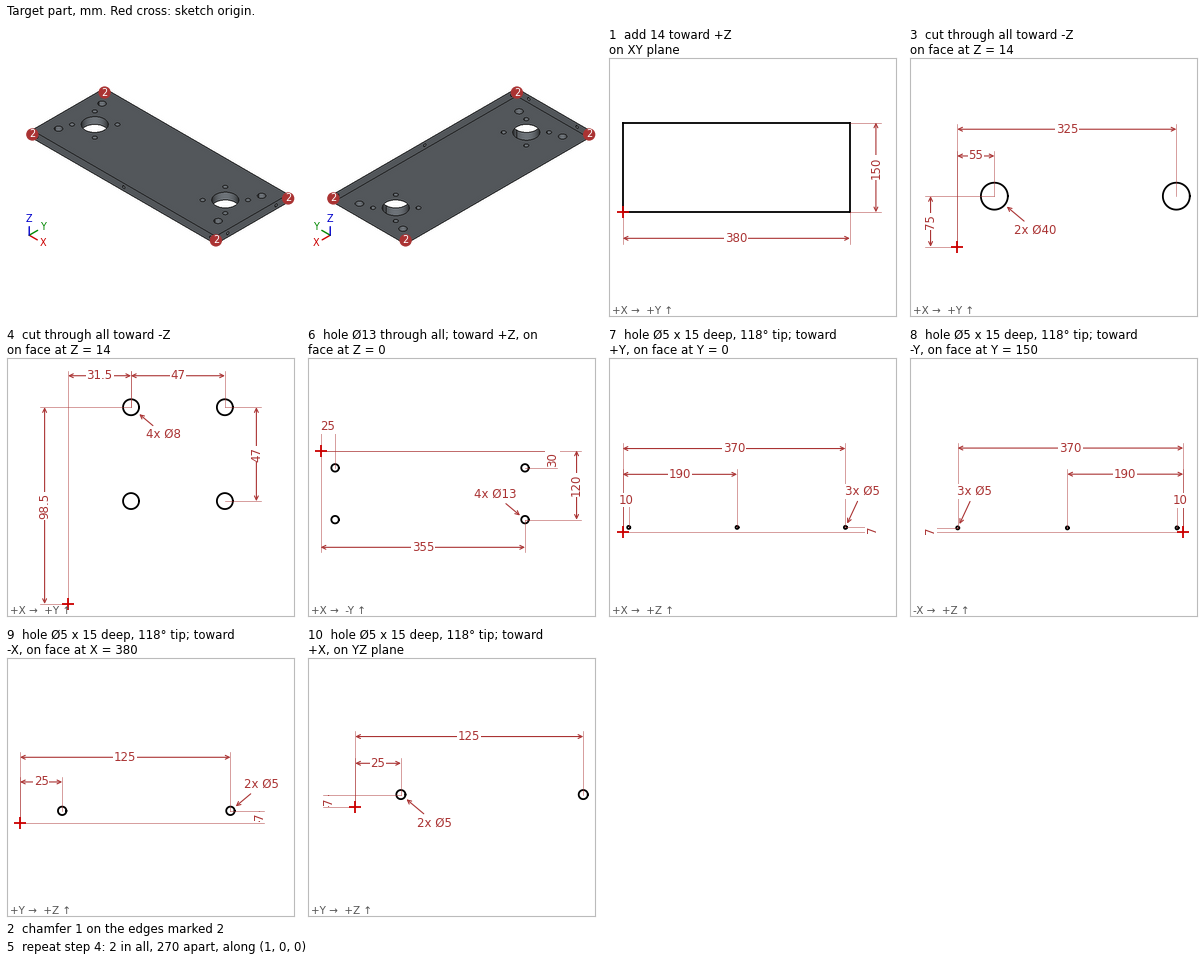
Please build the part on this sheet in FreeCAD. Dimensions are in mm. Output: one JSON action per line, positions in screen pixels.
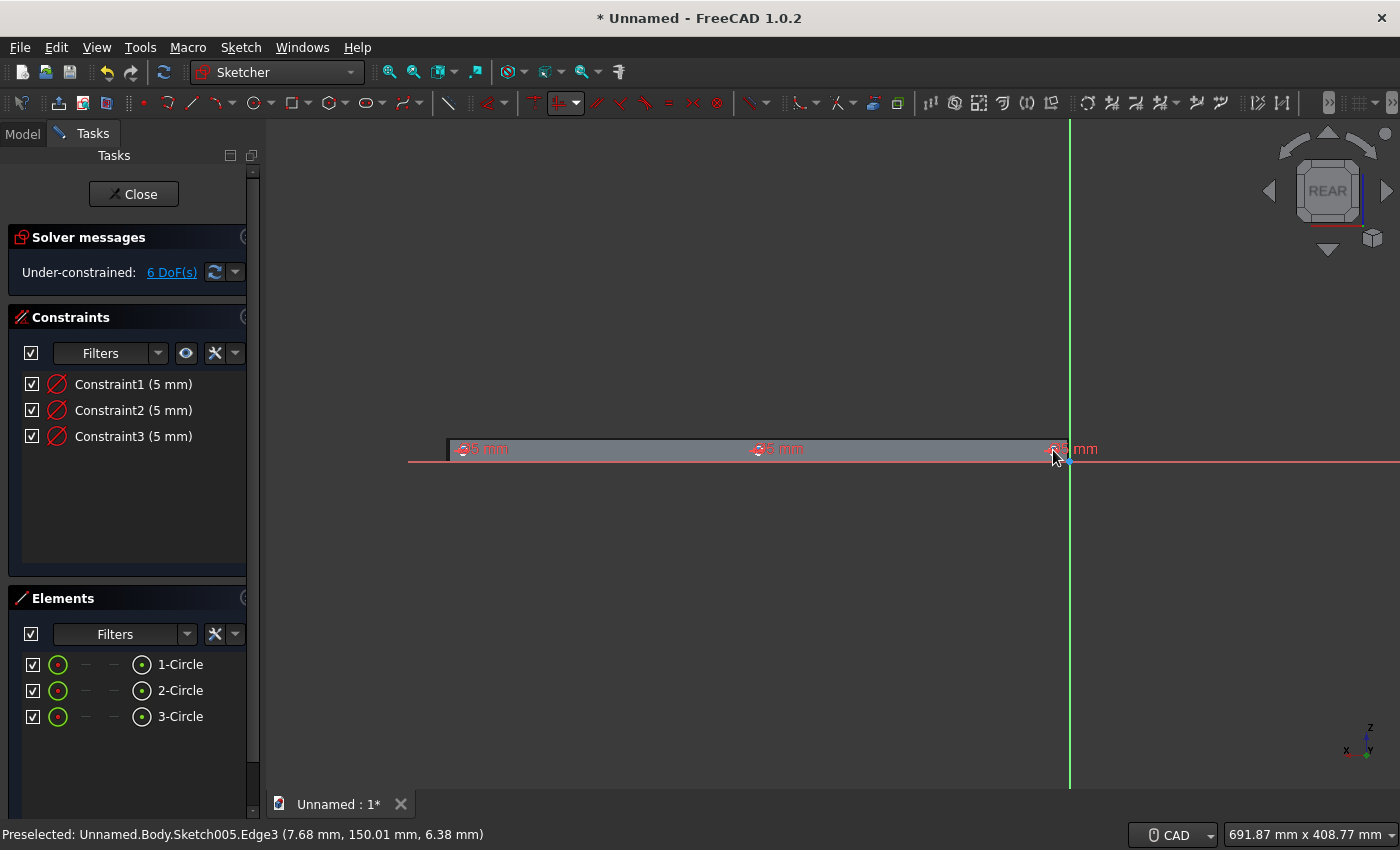
{"action": "left_click", "coordinate": [463, 451]}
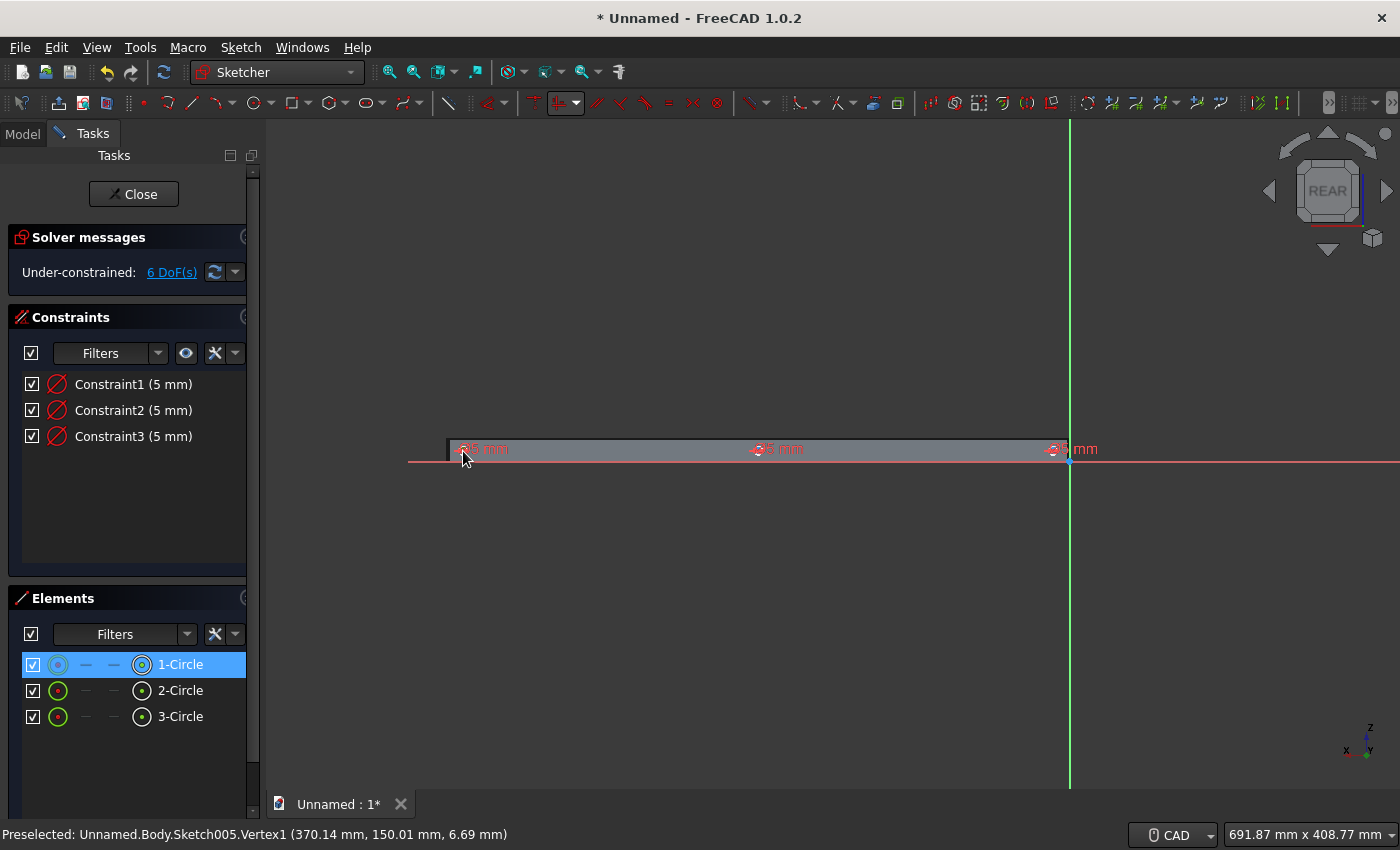
{"action": "left_click", "coordinate": [759, 451]}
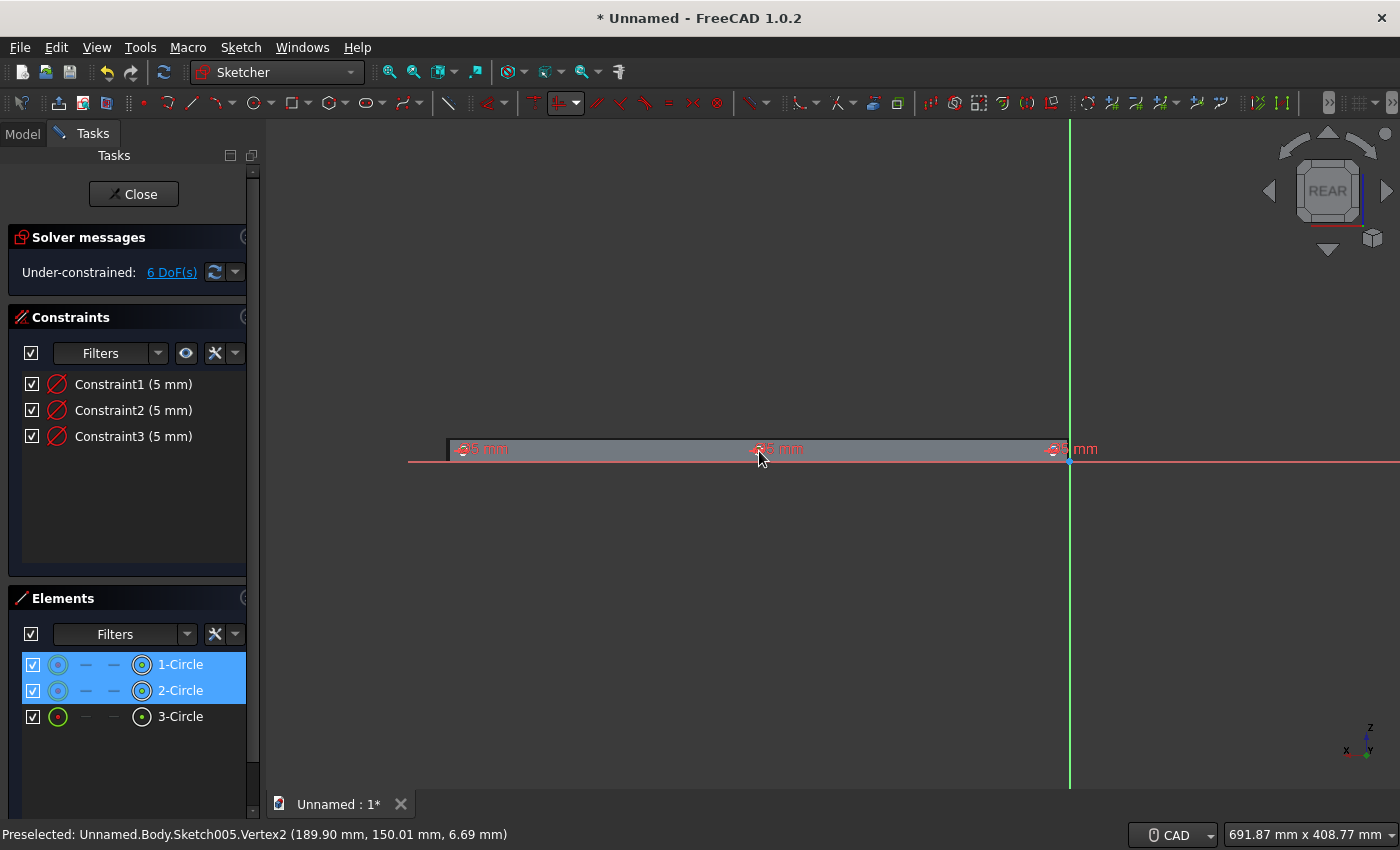
{"action": "key", "text": "h"}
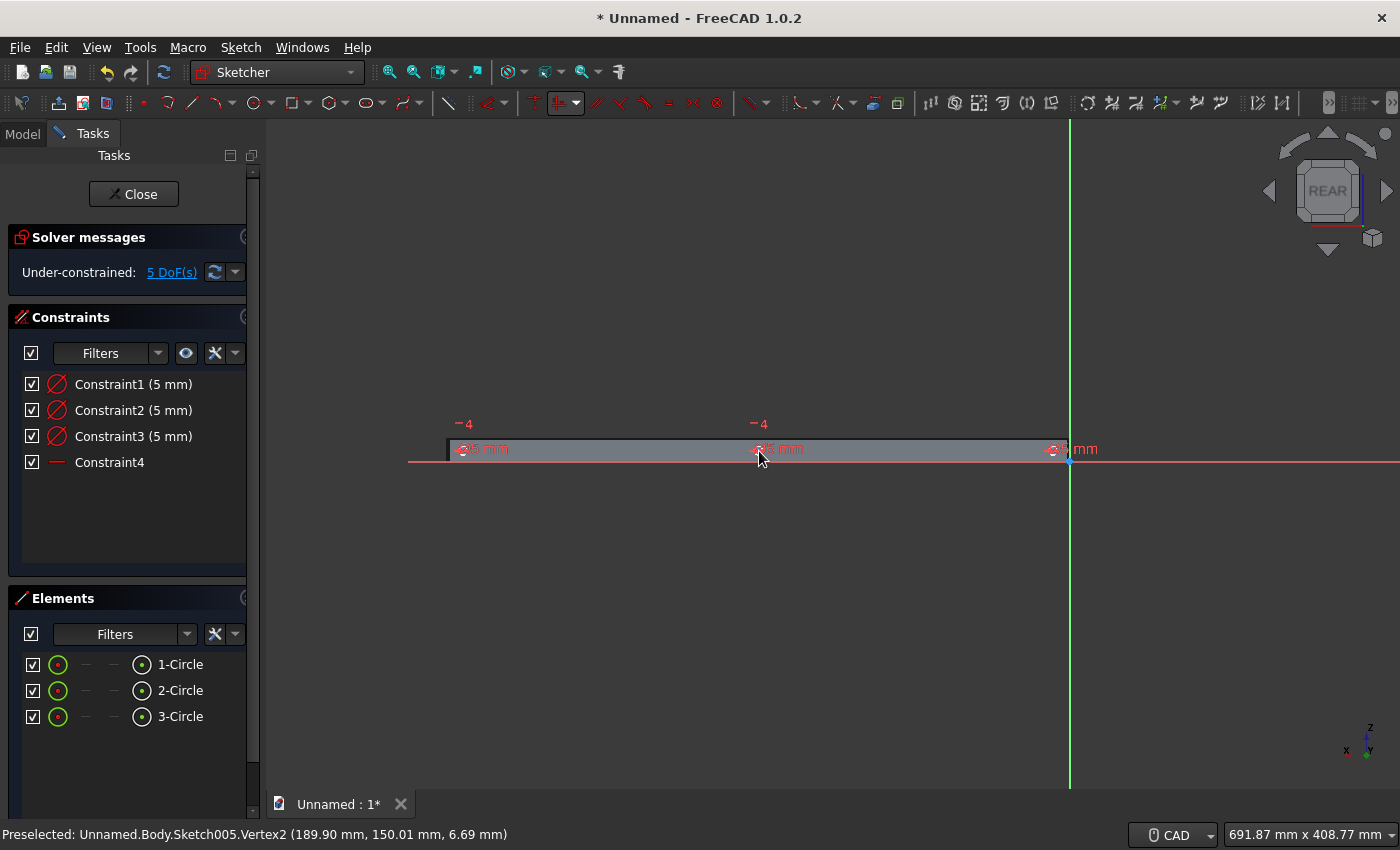
{"action": "left_click", "coordinate": [759, 451]}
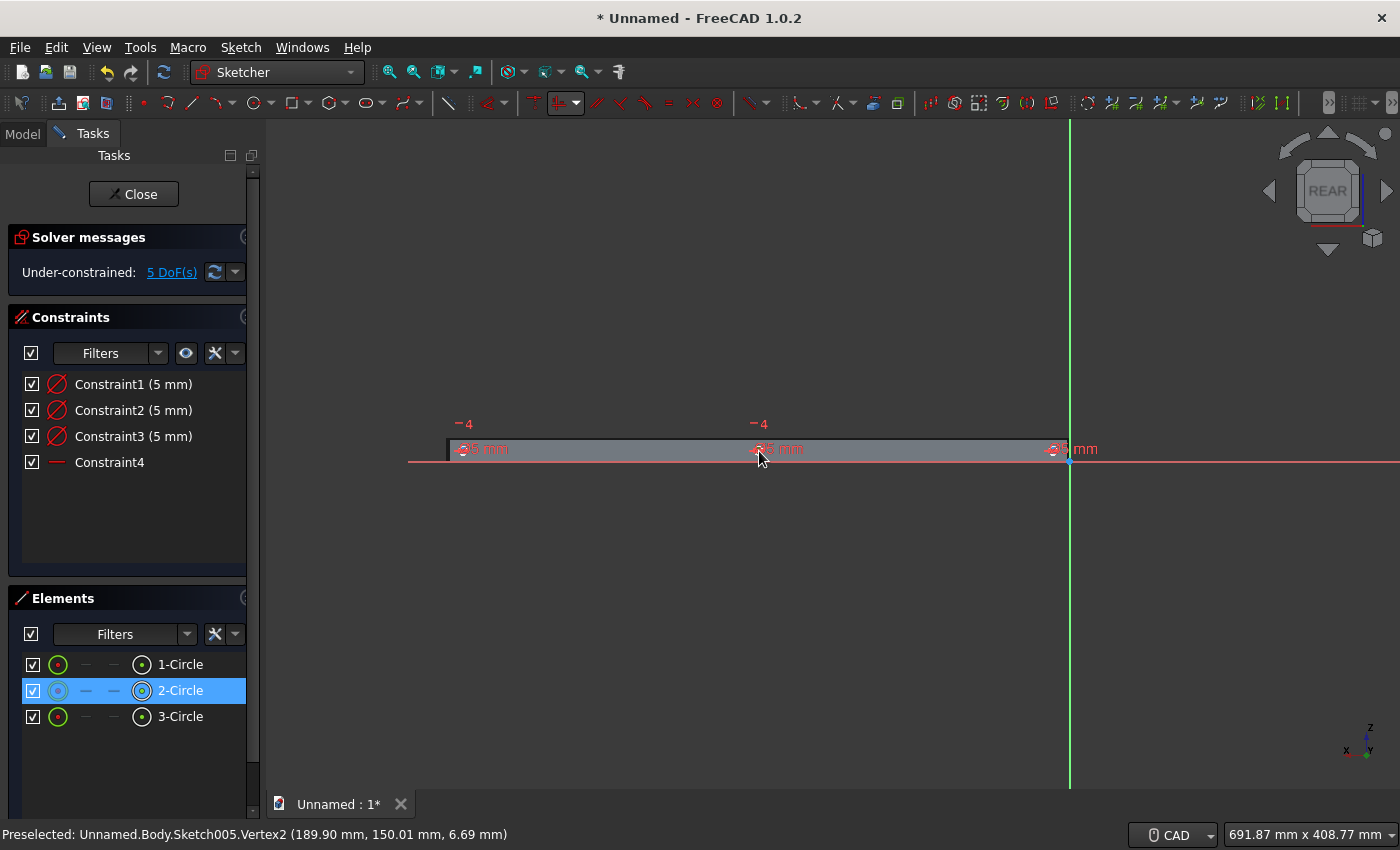
{"action": "left_click", "coordinate": [1053, 451]}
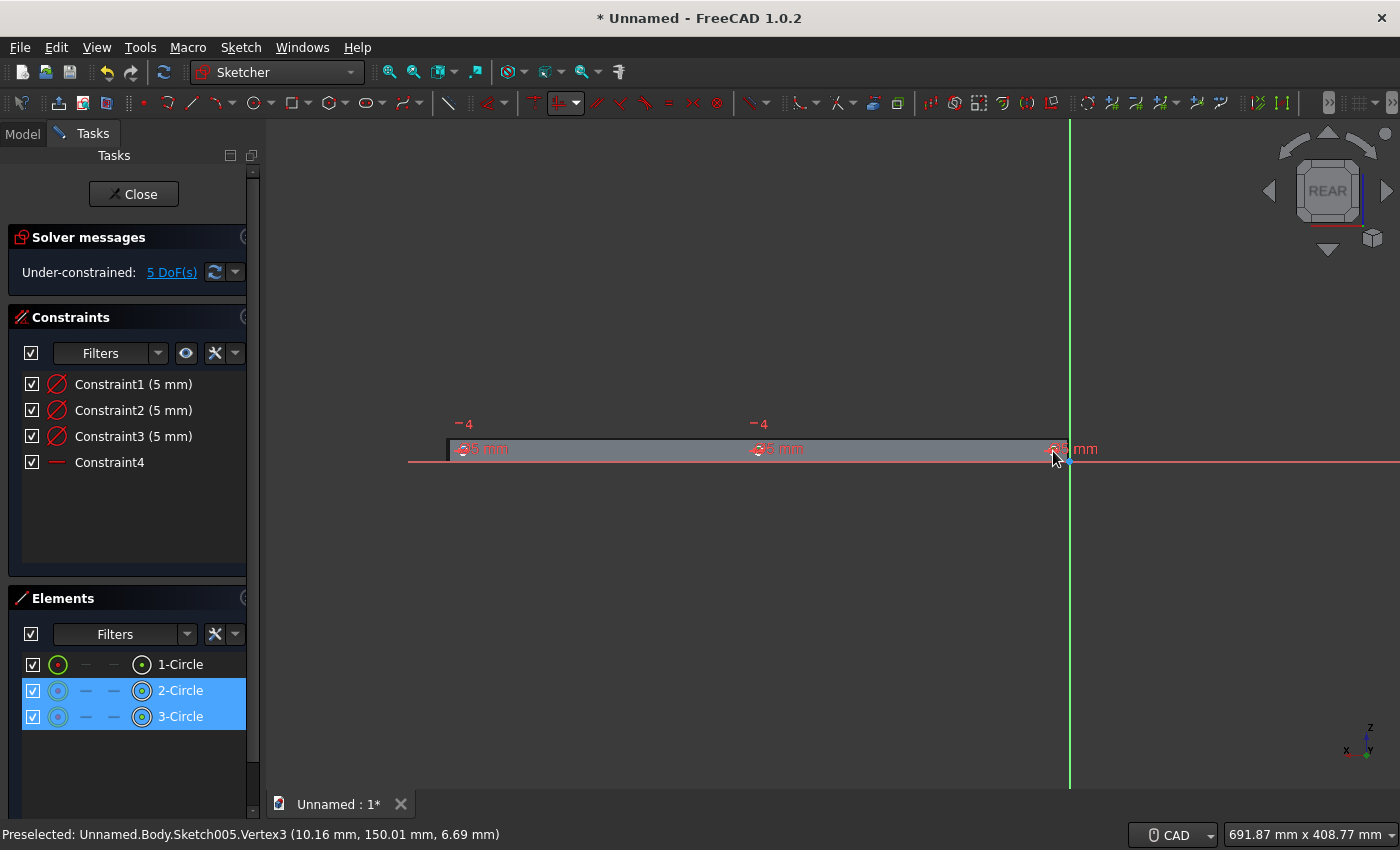
{"action": "key", "text": "h"}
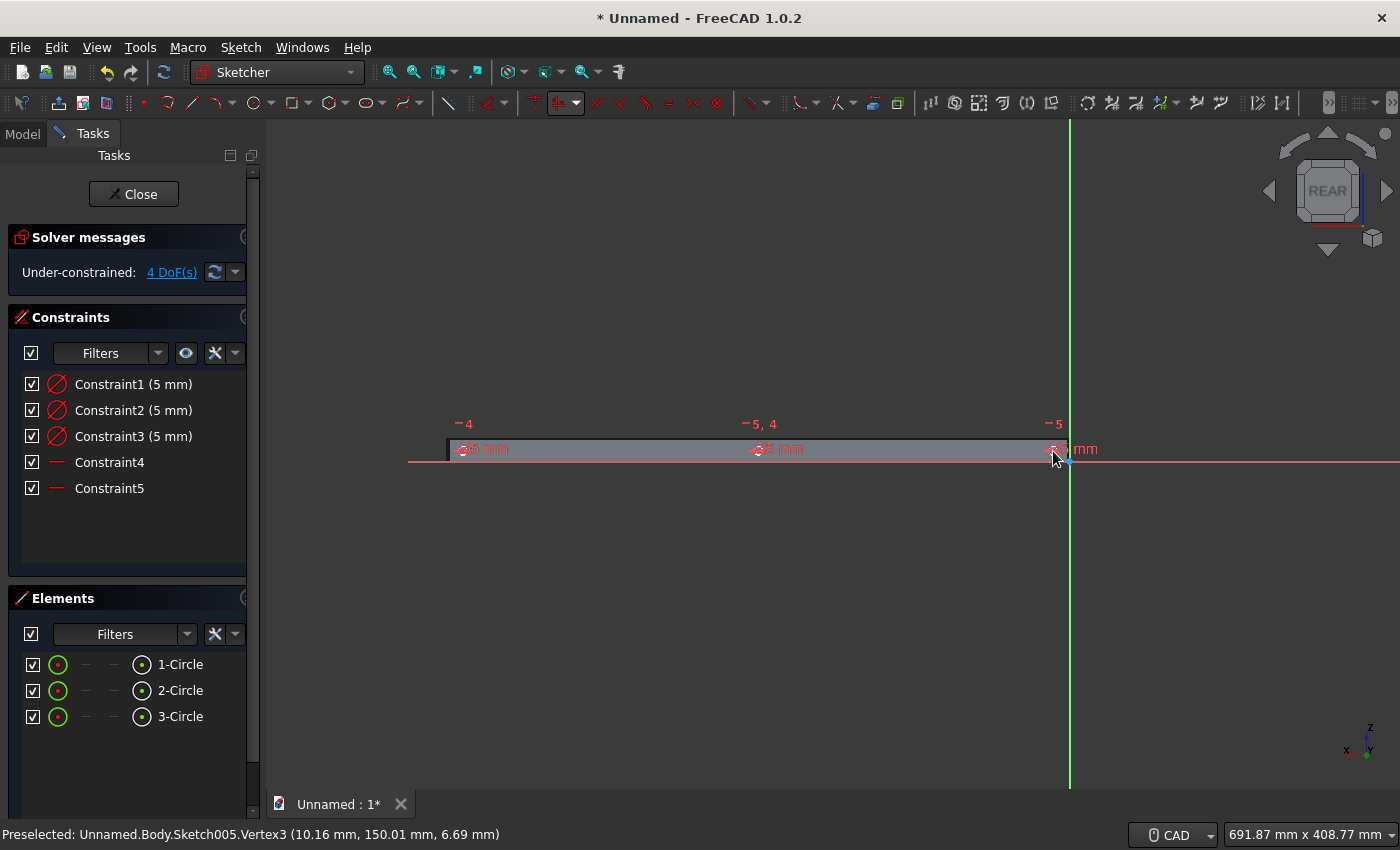
{"action": "key", "text": "d"}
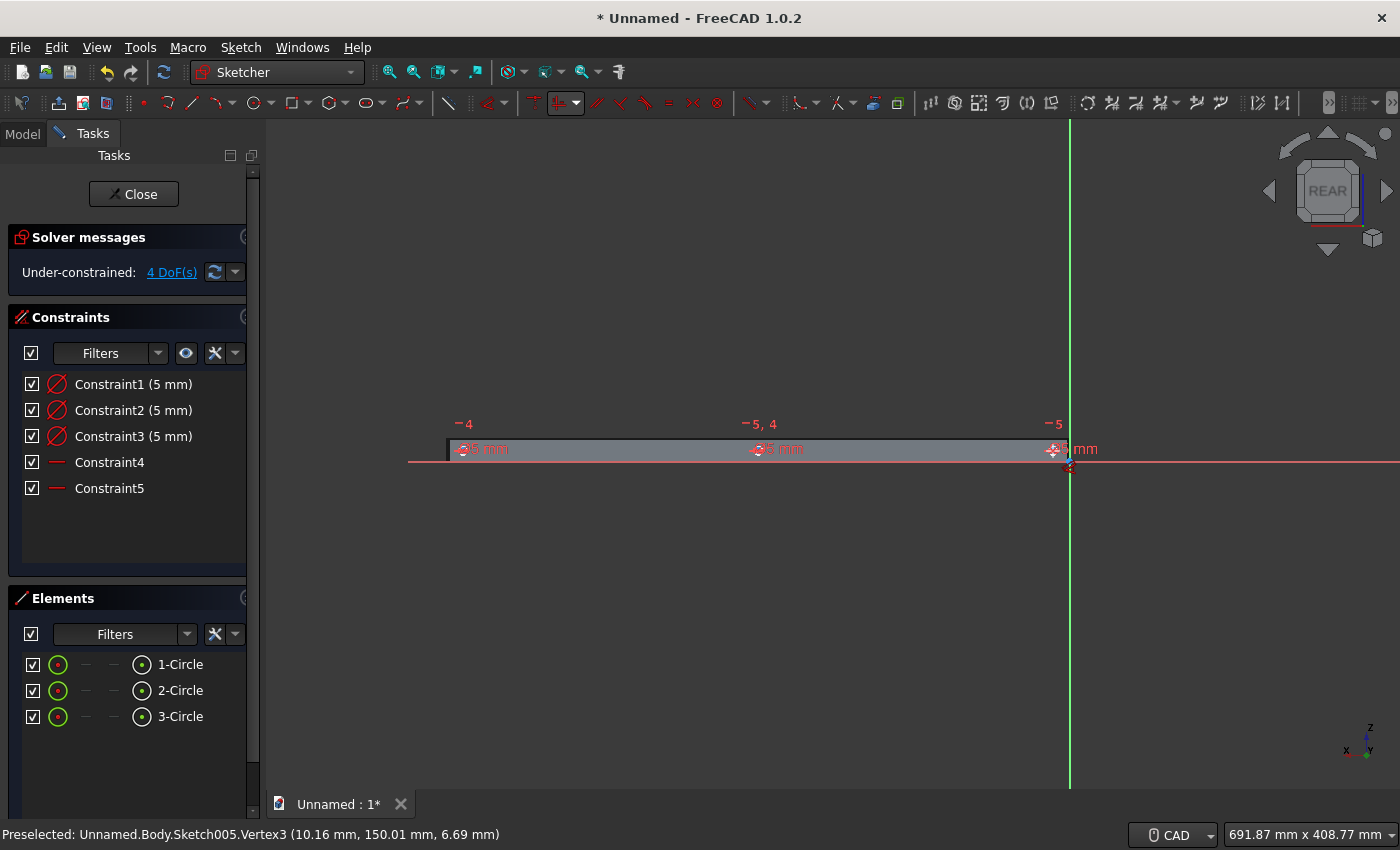
{"action": "scroll", "coordinate": [463, 451], "scroll_direction": "up", "scroll_amount": 7}